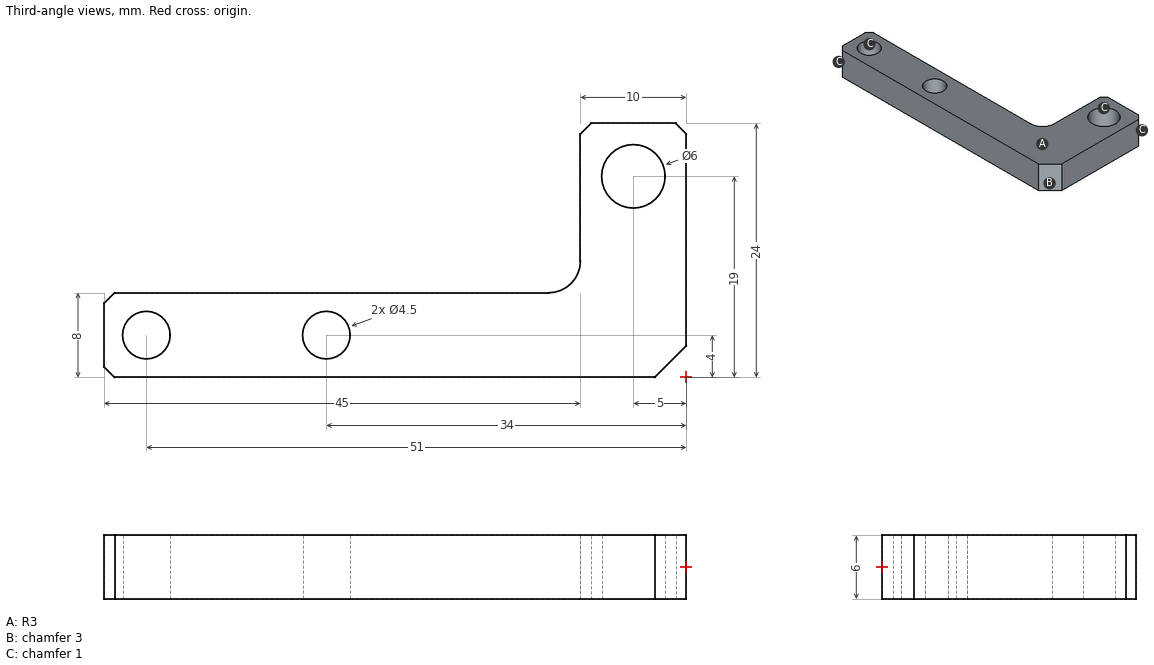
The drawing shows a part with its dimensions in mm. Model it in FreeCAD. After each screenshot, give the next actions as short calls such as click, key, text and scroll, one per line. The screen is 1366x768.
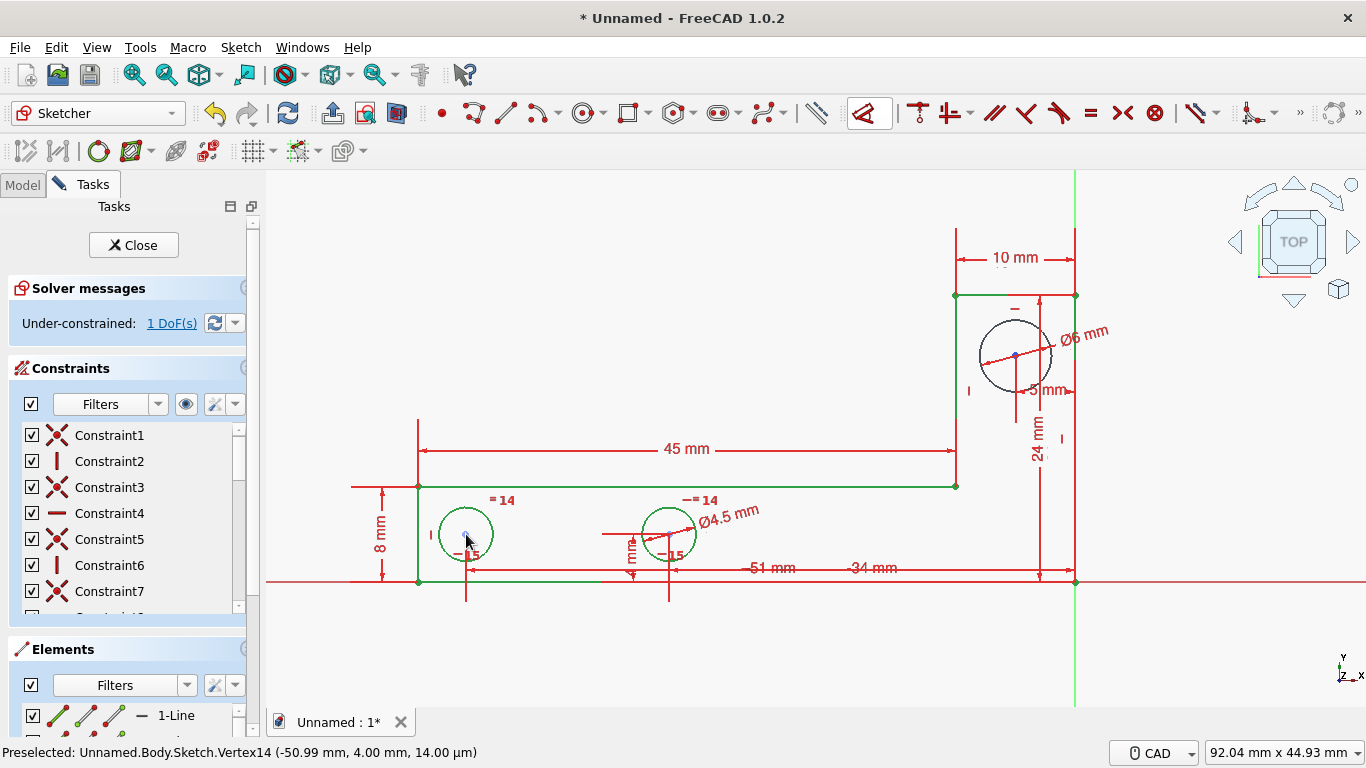
click(1016, 356)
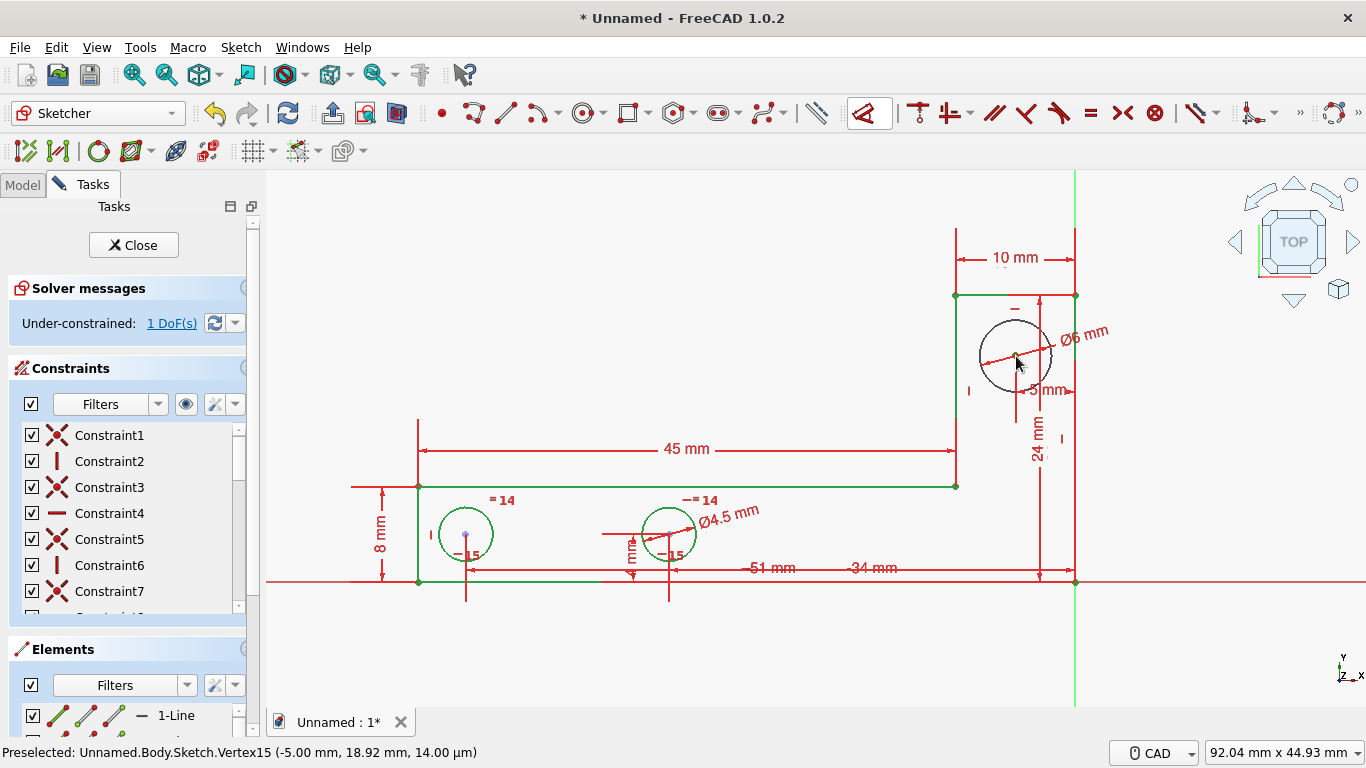
key(i)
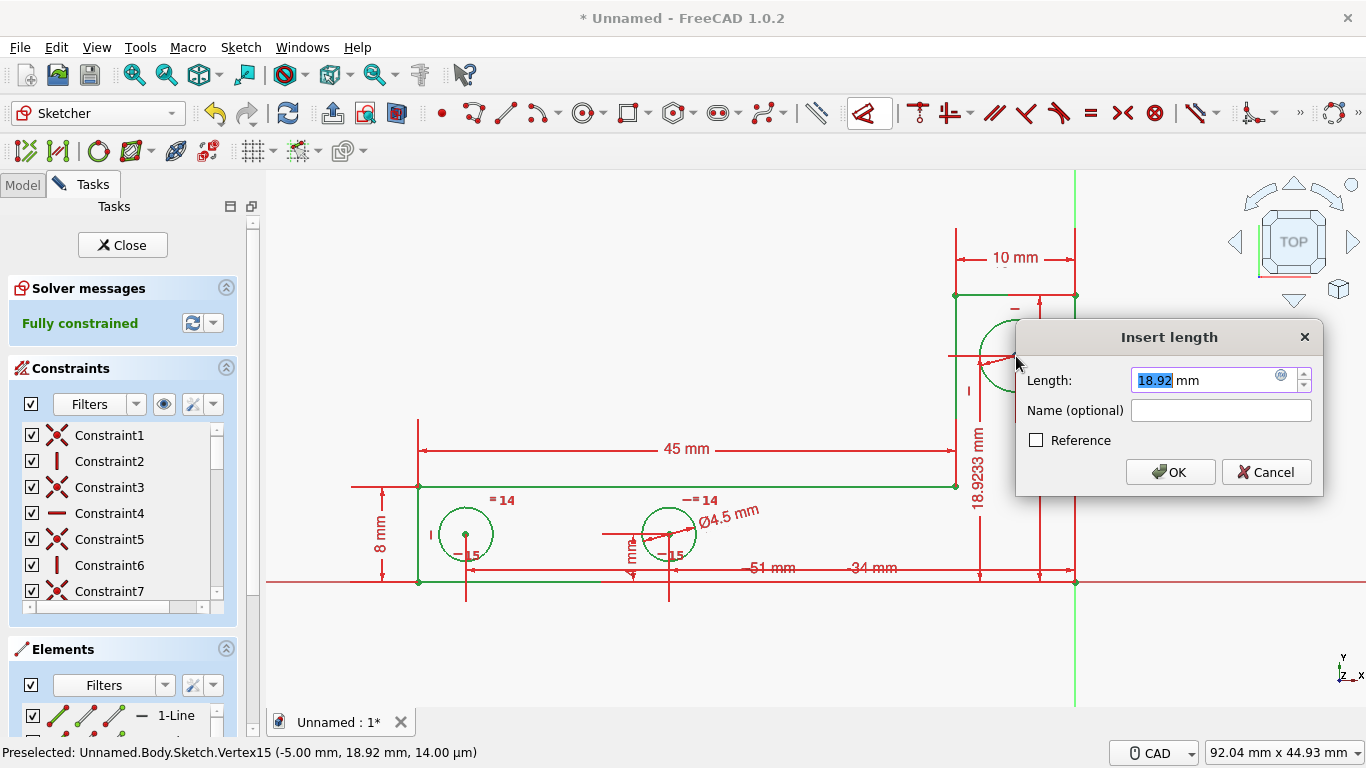
text(19)
key(Return)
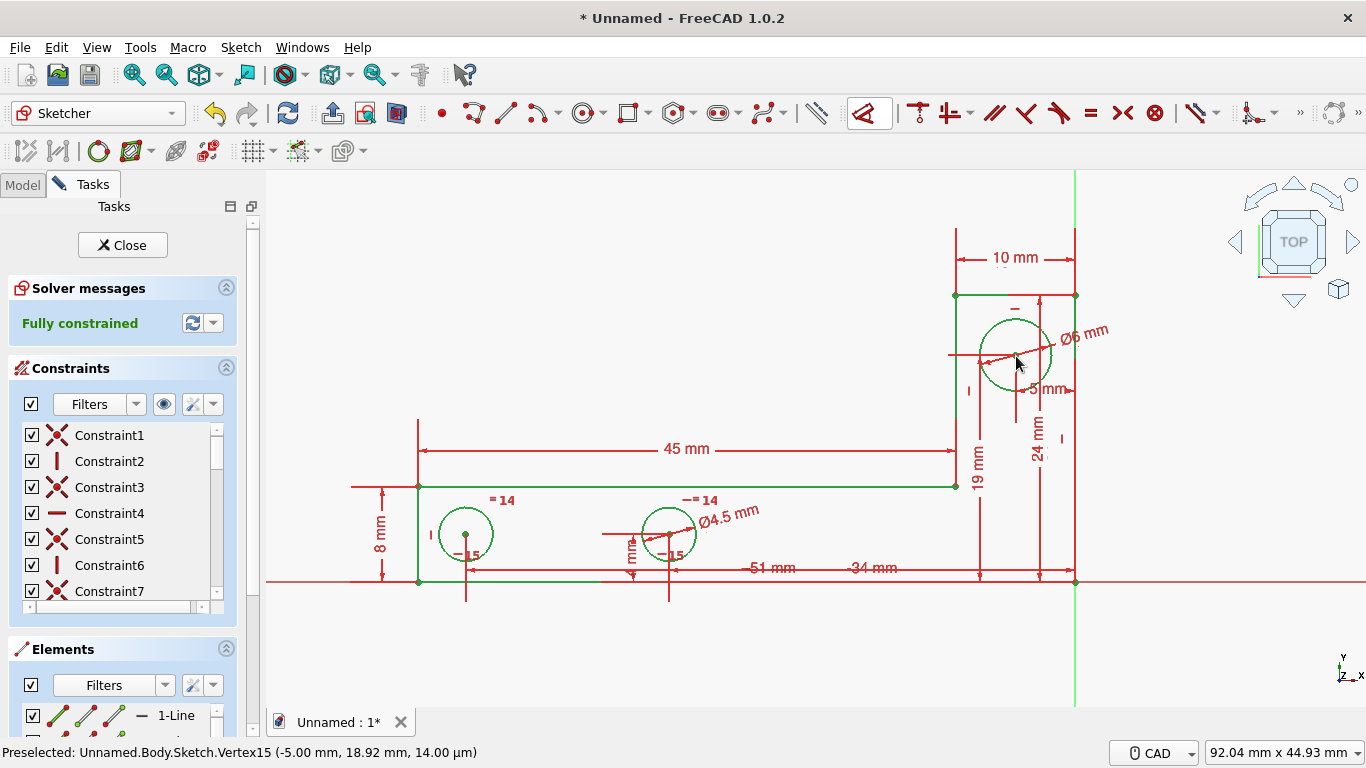
click(123, 245)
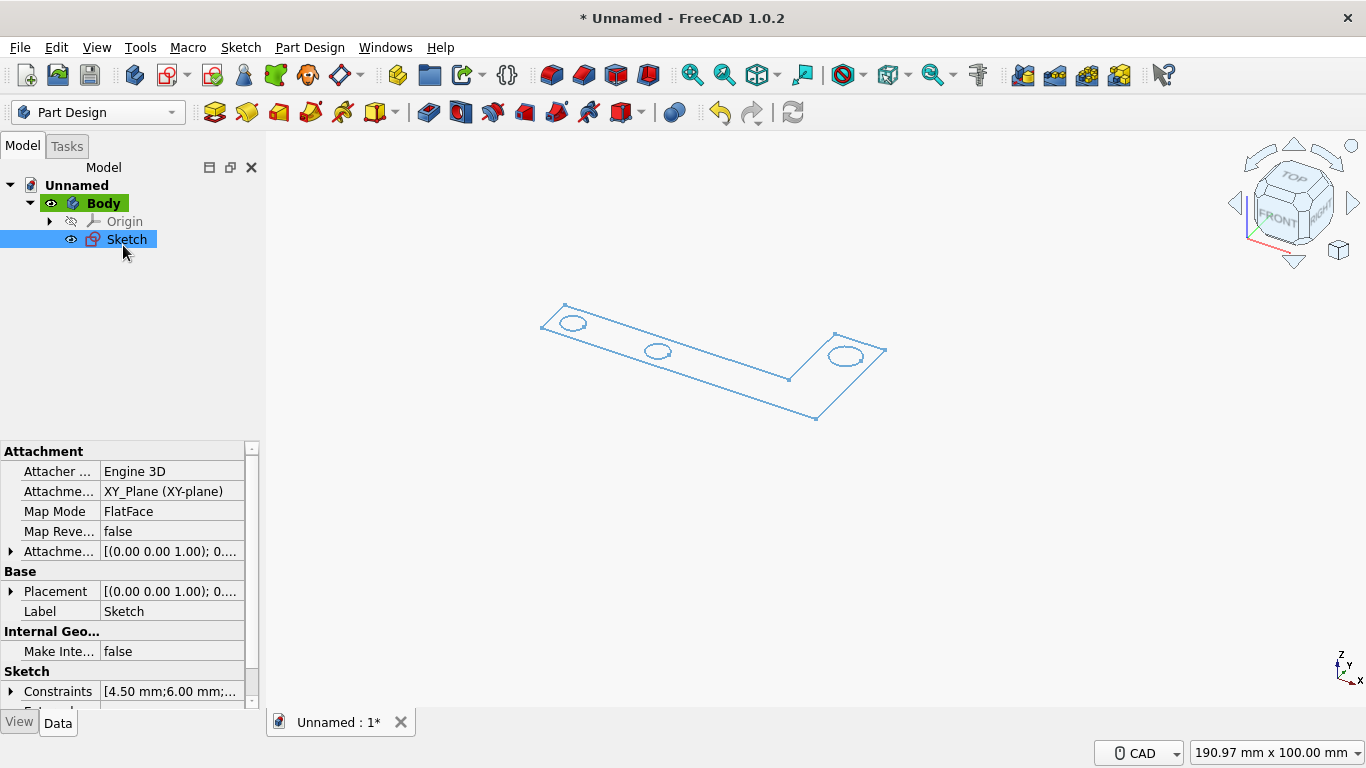
click(216, 112)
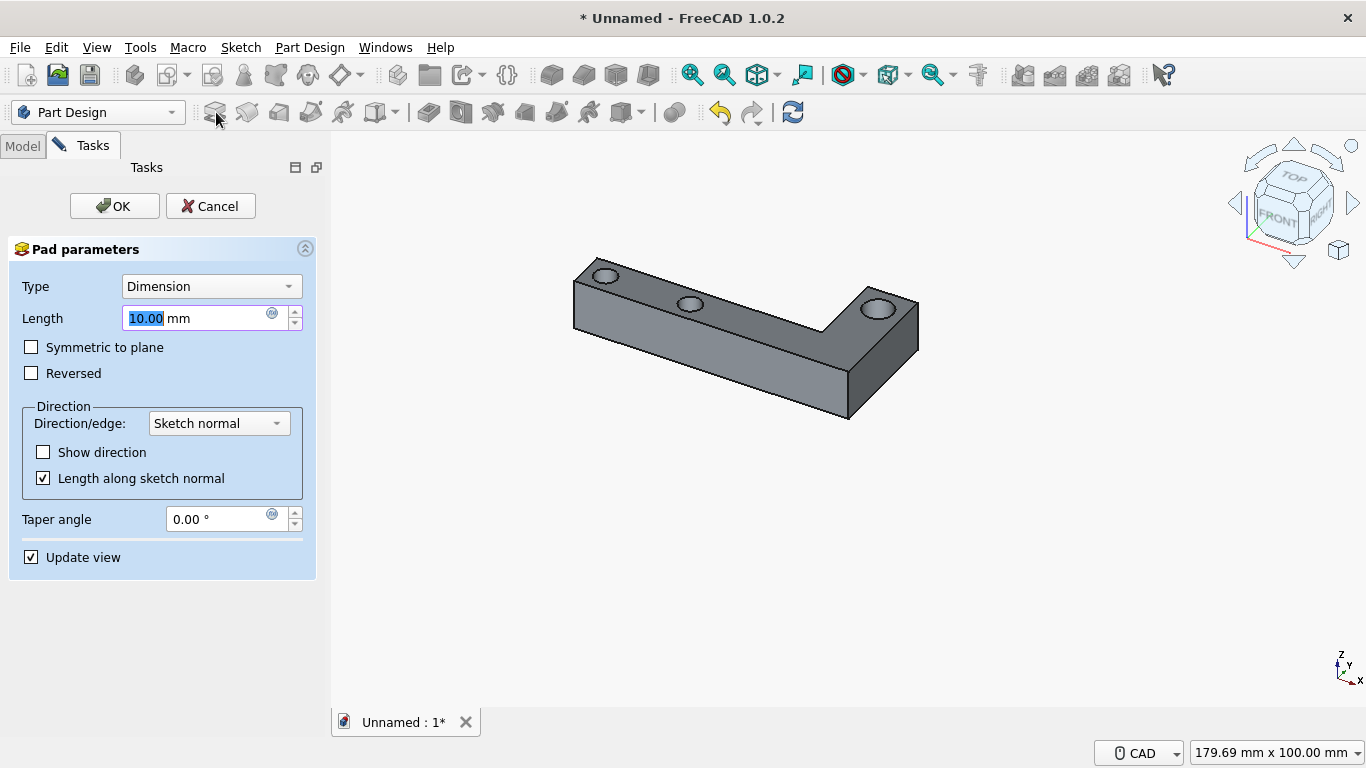
text(6)
key(Tab)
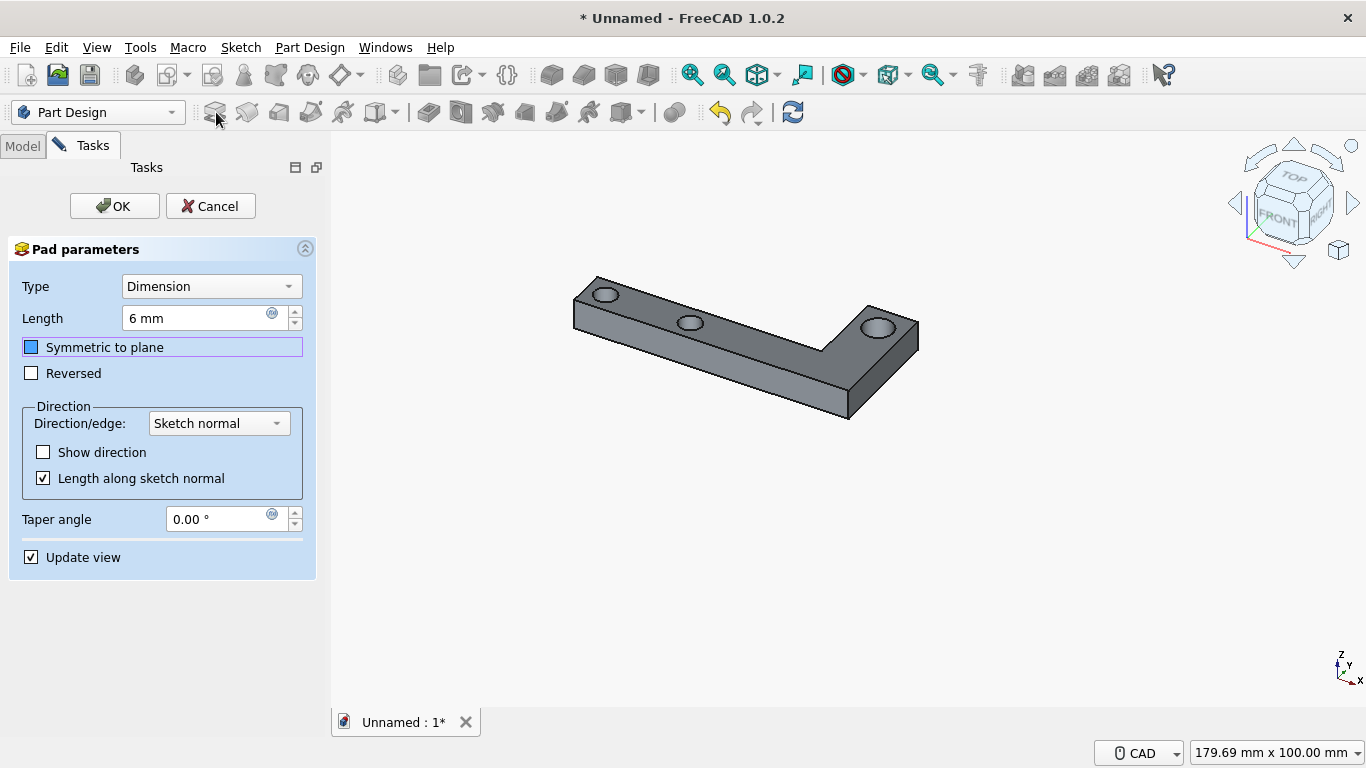
click(30, 347)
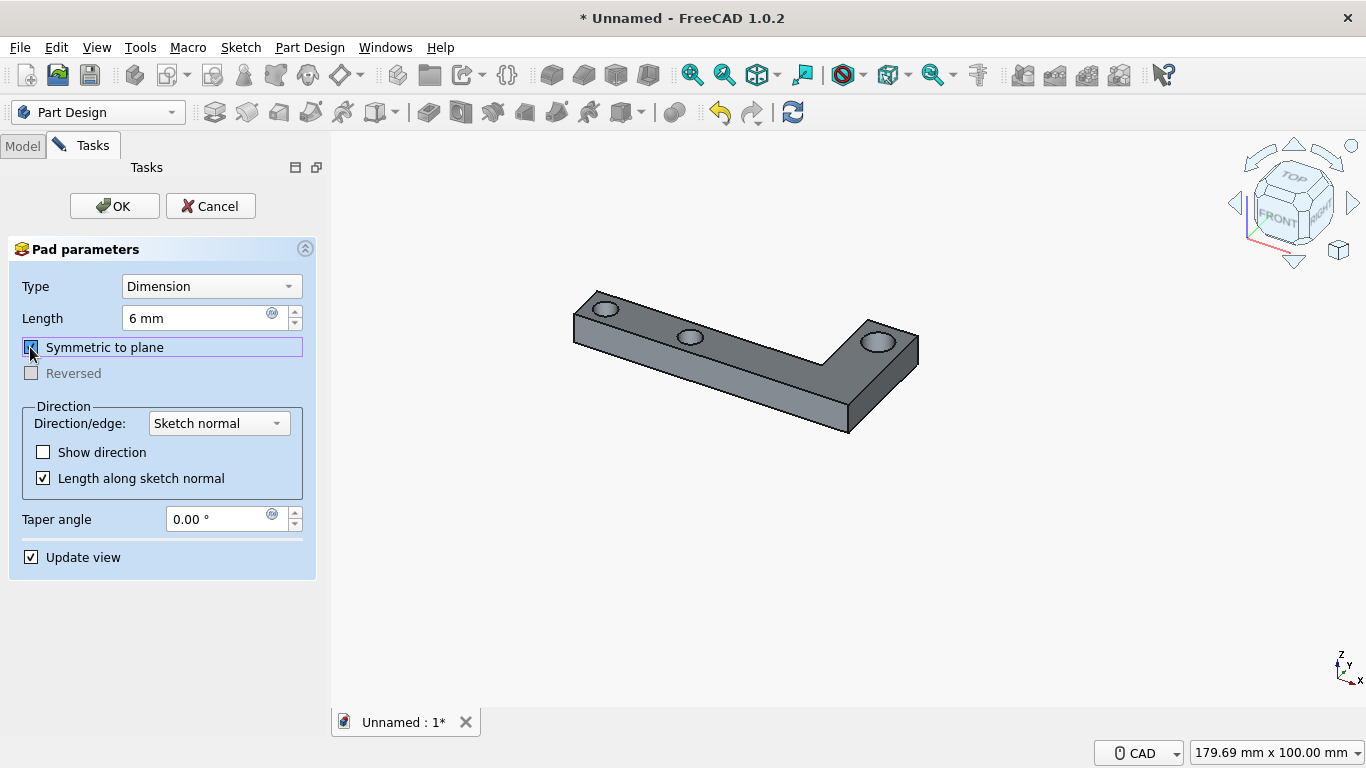
click(115, 206)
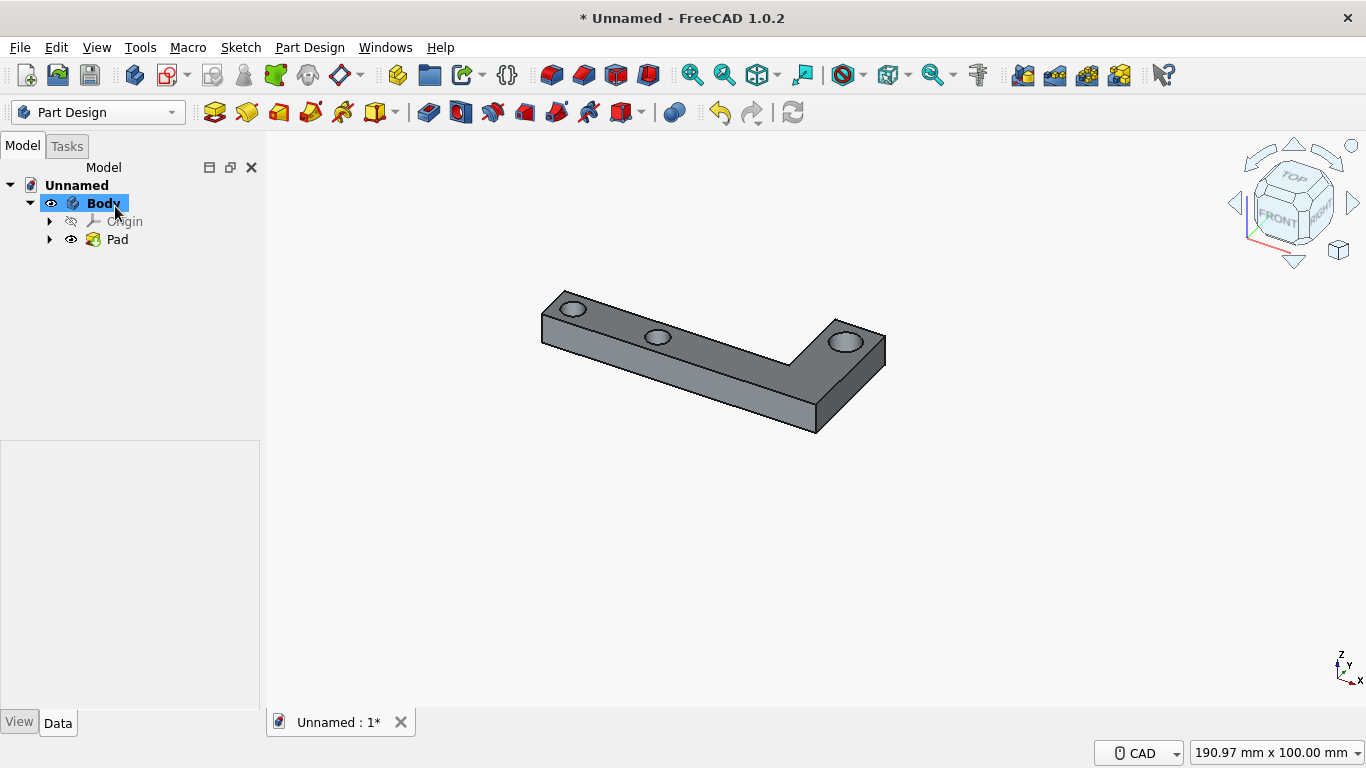
click(694, 76)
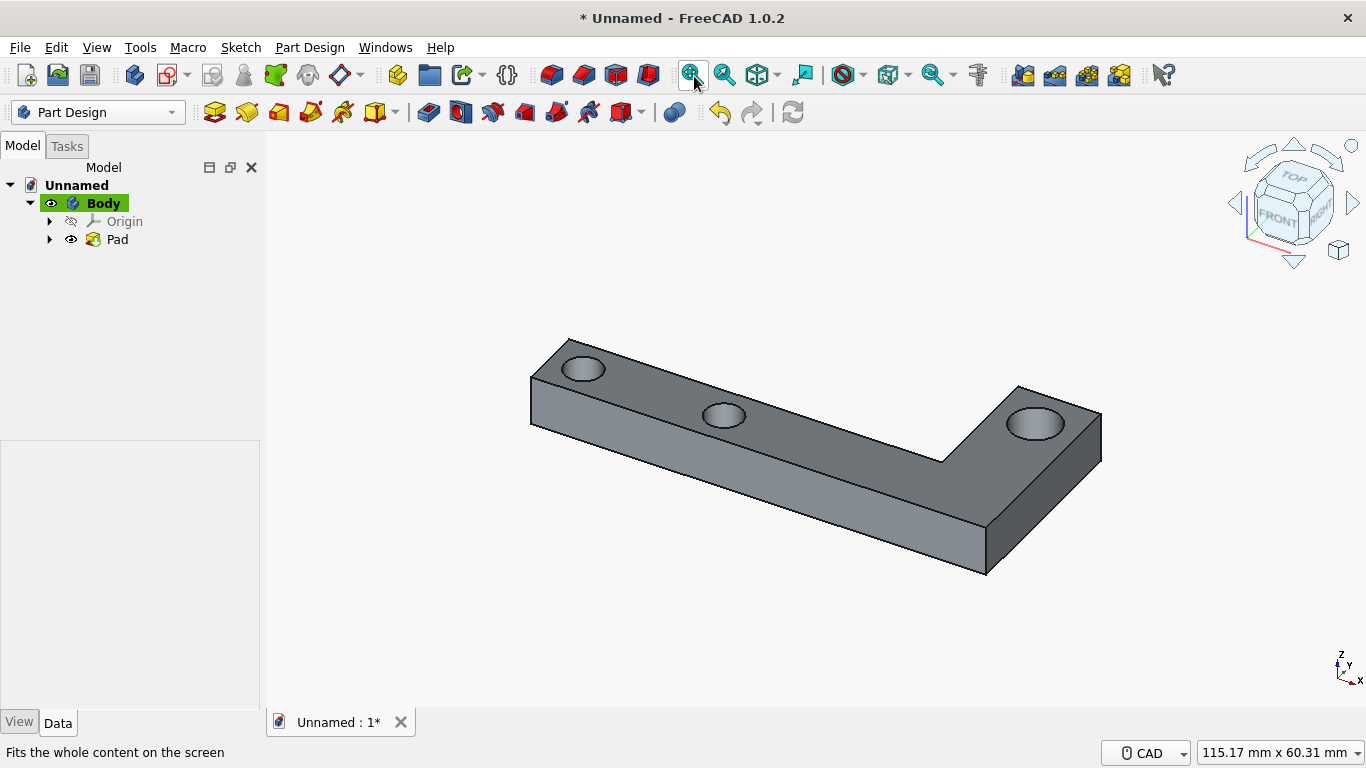
key(0)